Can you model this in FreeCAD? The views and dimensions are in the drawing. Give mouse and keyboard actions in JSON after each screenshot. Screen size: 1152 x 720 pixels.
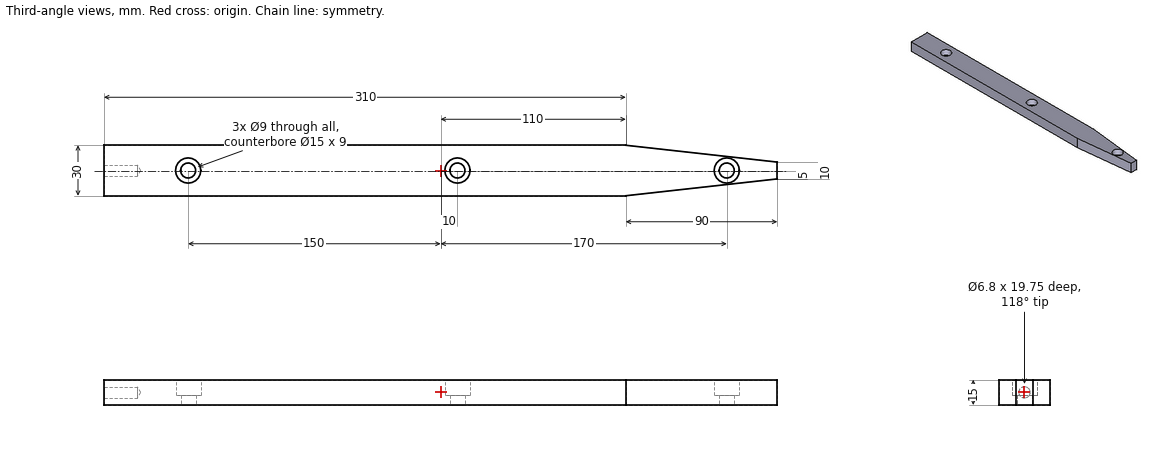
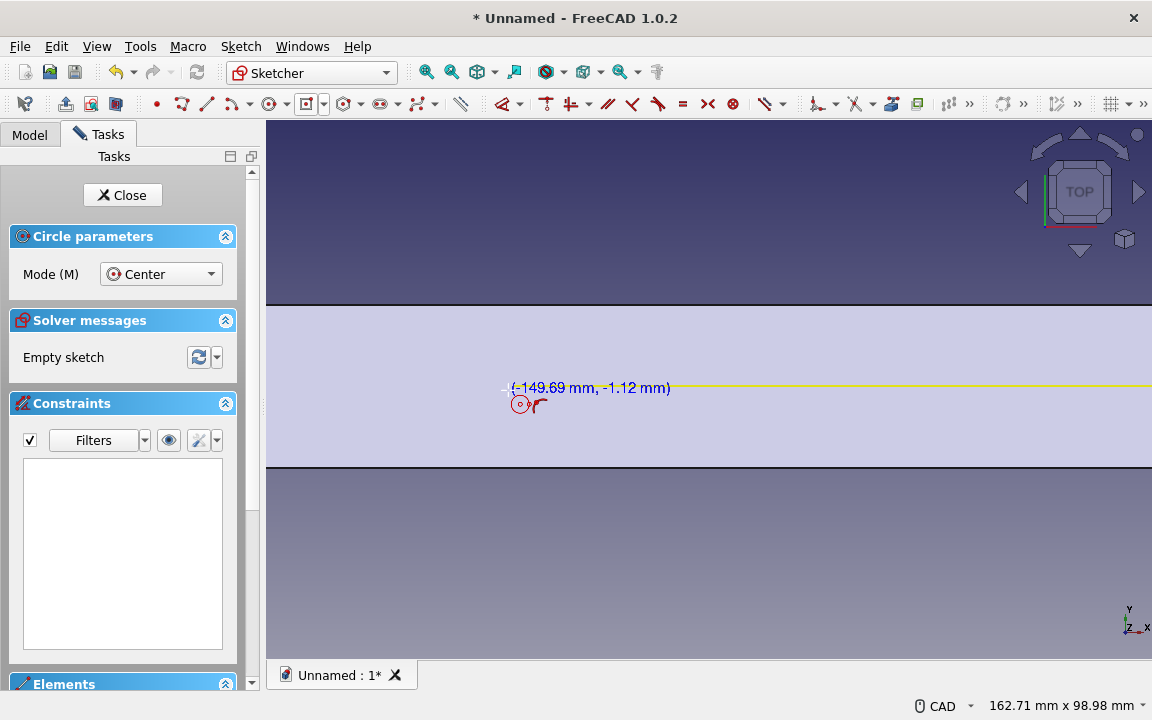
{"action": "scroll", "coordinate": [323, 391], "scroll_direction": "down", "scroll_amount": 6}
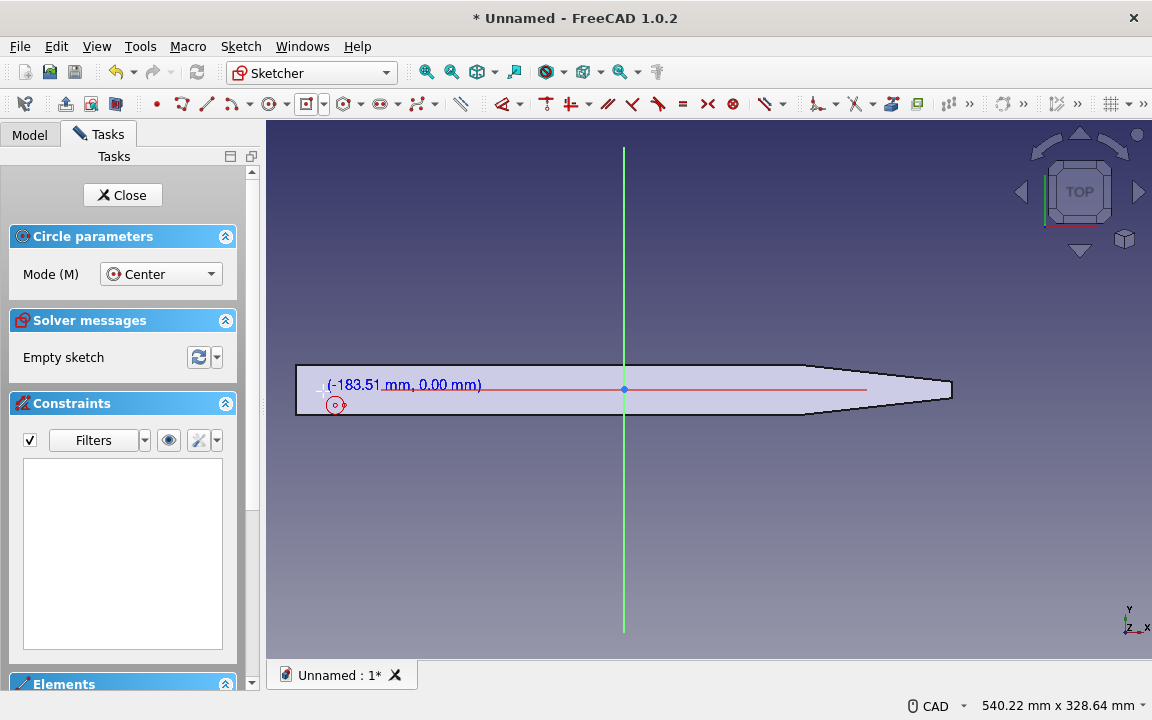
{"action": "left_click", "coordinate": [378, 390]}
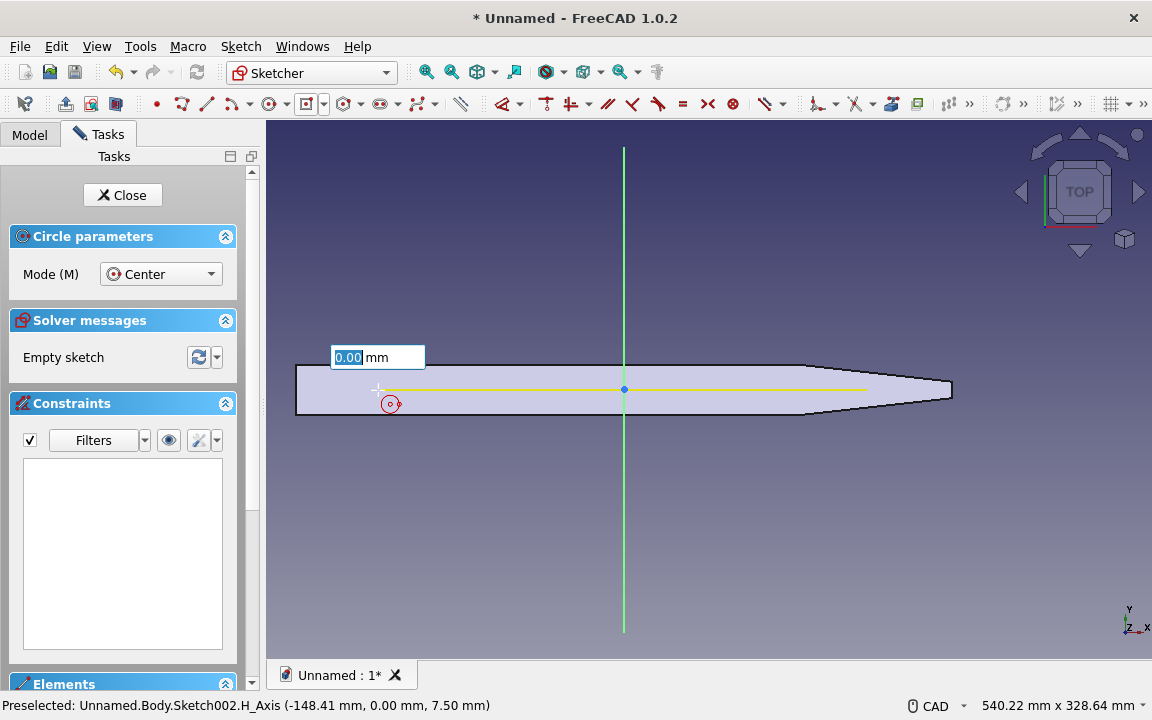
{"action": "scroll", "coordinate": [375, 397], "scroll_direction": "up", "scroll_amount": 5}
{"action": "mouse_move", "coordinate": [376, 396]}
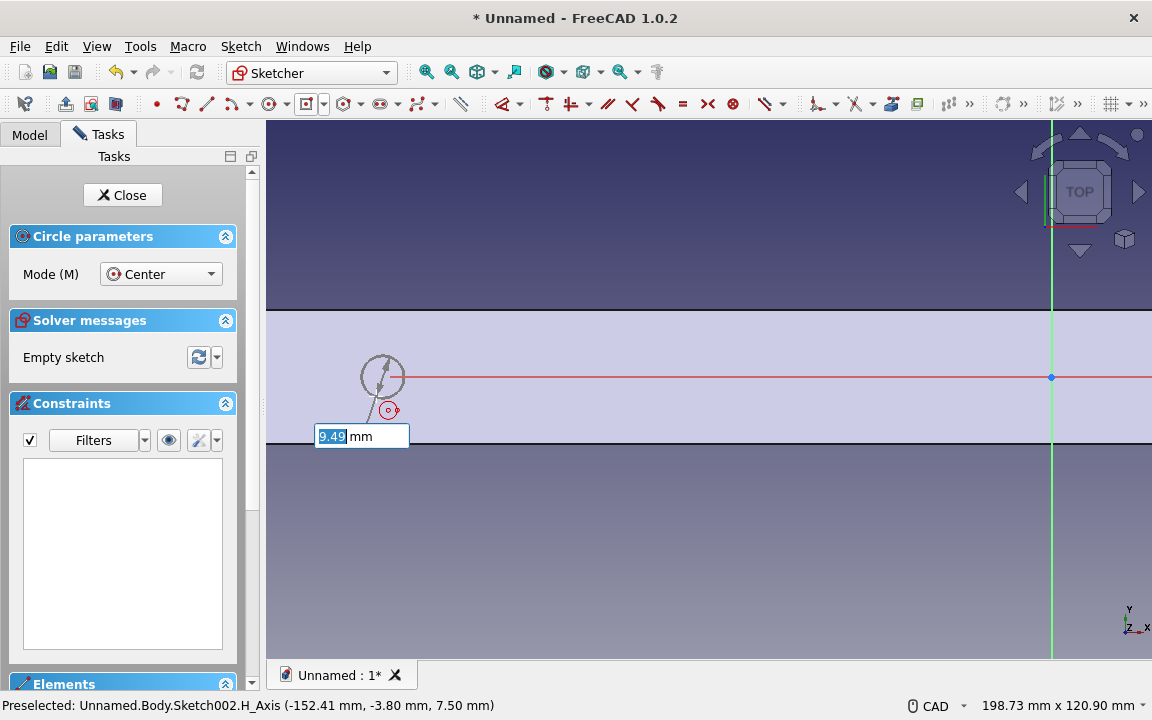
{"action": "type", "text": "9"}
{"action": "key", "text": "Return"}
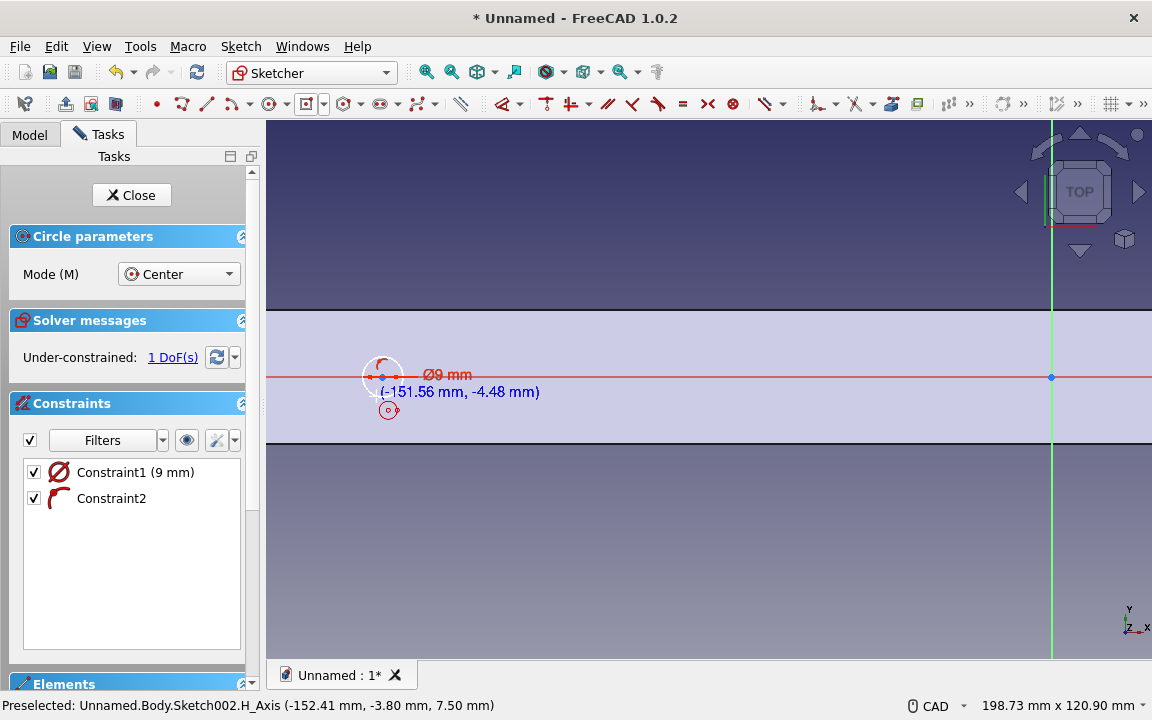
{"action": "scroll", "coordinate": [375, 397], "scroll_direction": "down", "scroll_amount": 5}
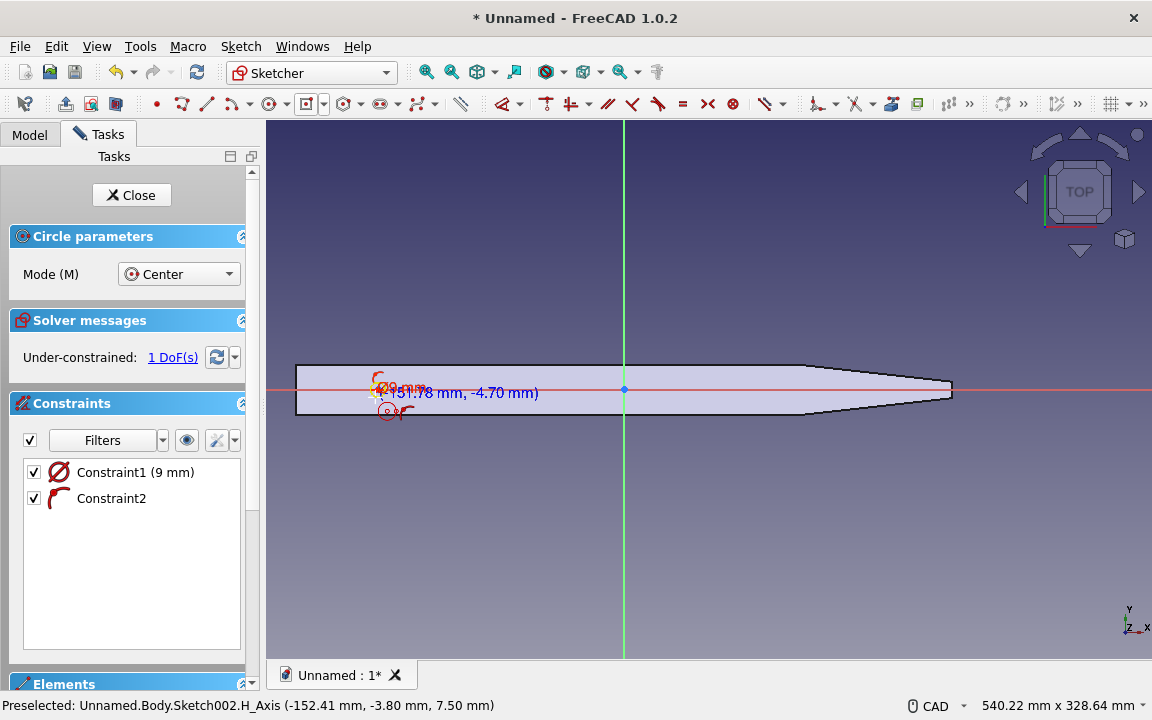
{"action": "scroll", "coordinate": [903, 390], "scroll_direction": "up", "scroll_amount": 6}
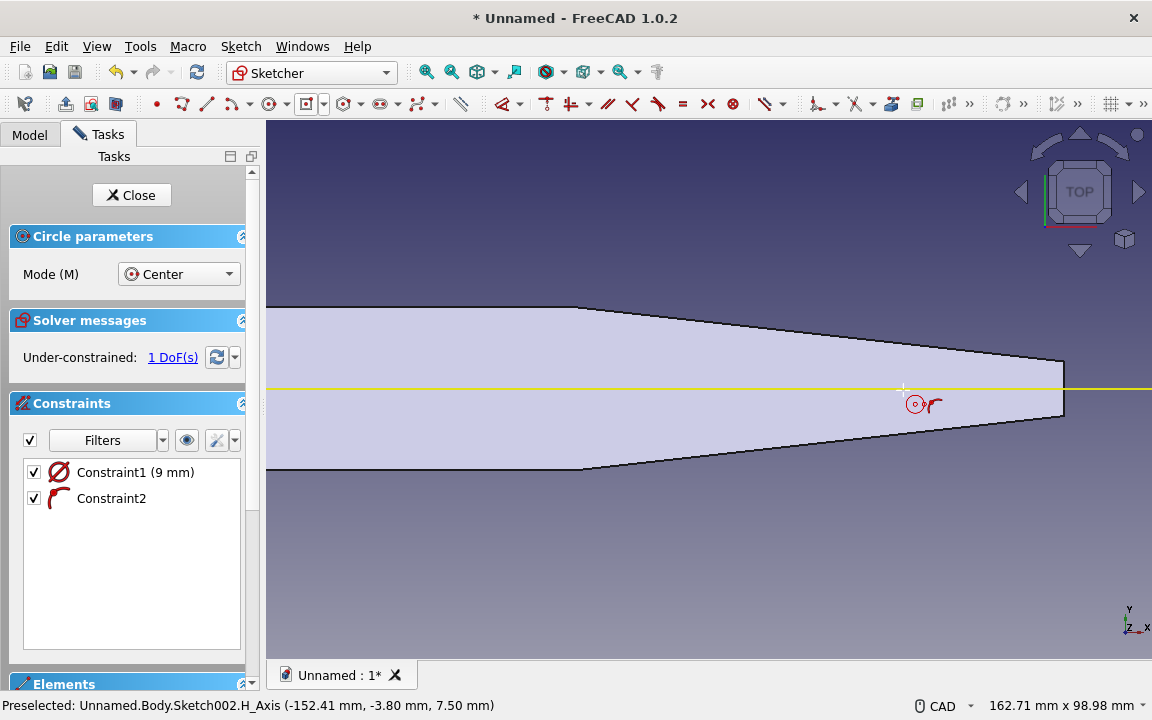
{"action": "scroll", "coordinate": [904, 390], "scroll_direction": "down", "scroll_amount": 6}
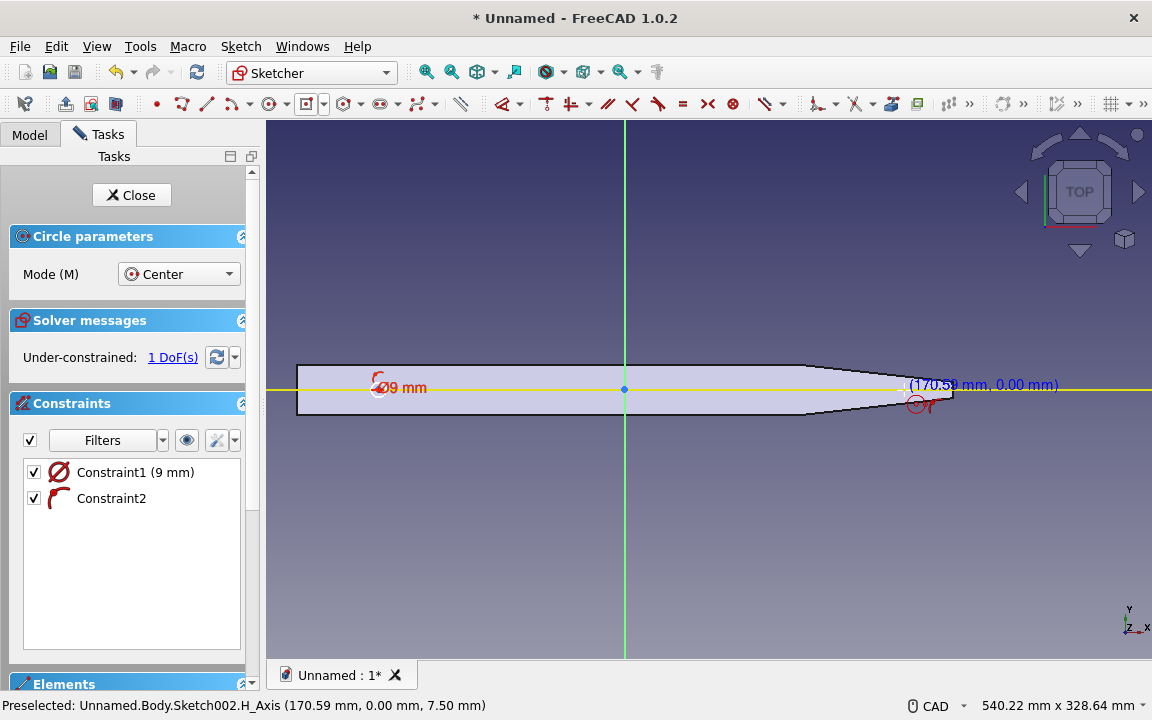
{"action": "left_click", "coordinate": [904, 390]}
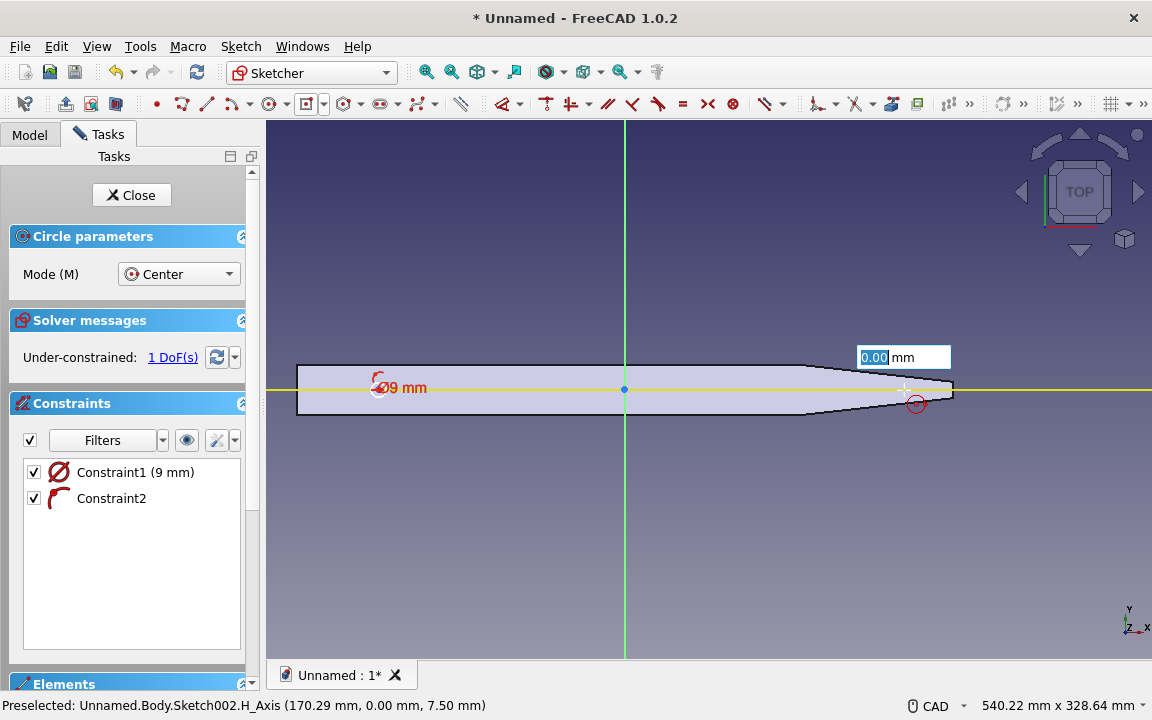
{"action": "scroll", "coordinate": [901, 397], "scroll_direction": "up", "scroll_amount": 5}
{"action": "mouse_move", "coordinate": [900, 396]}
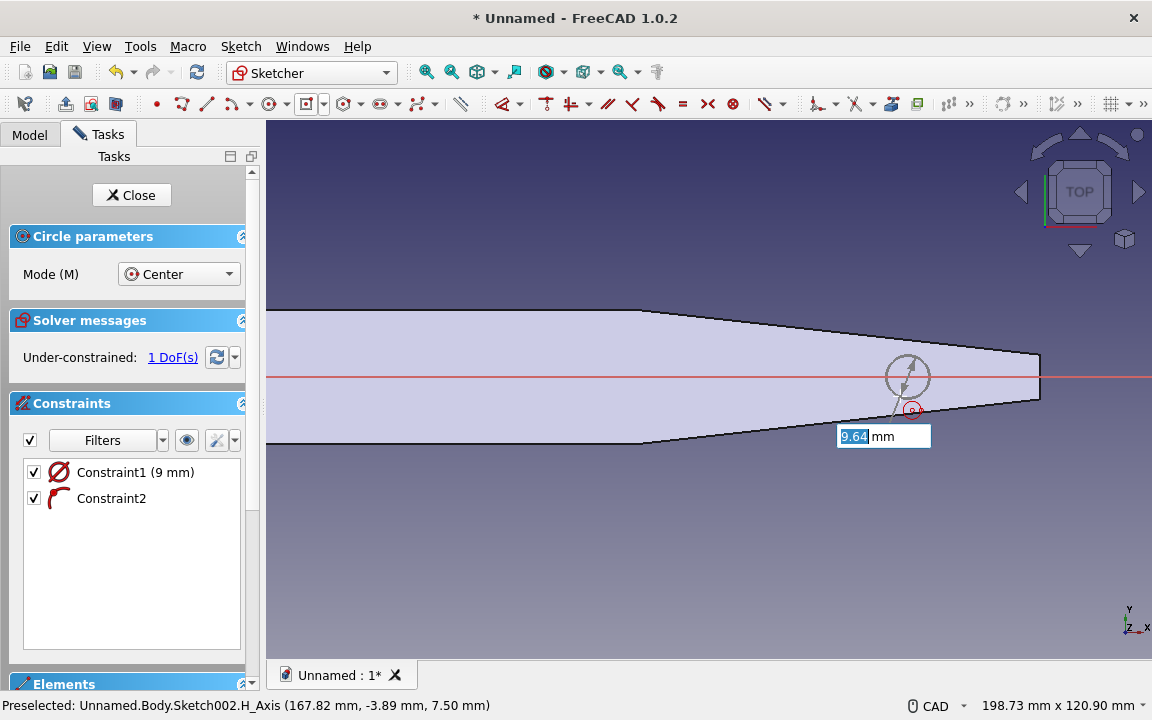
{"action": "type", "text": "9"}
{"action": "key", "text": "Return"}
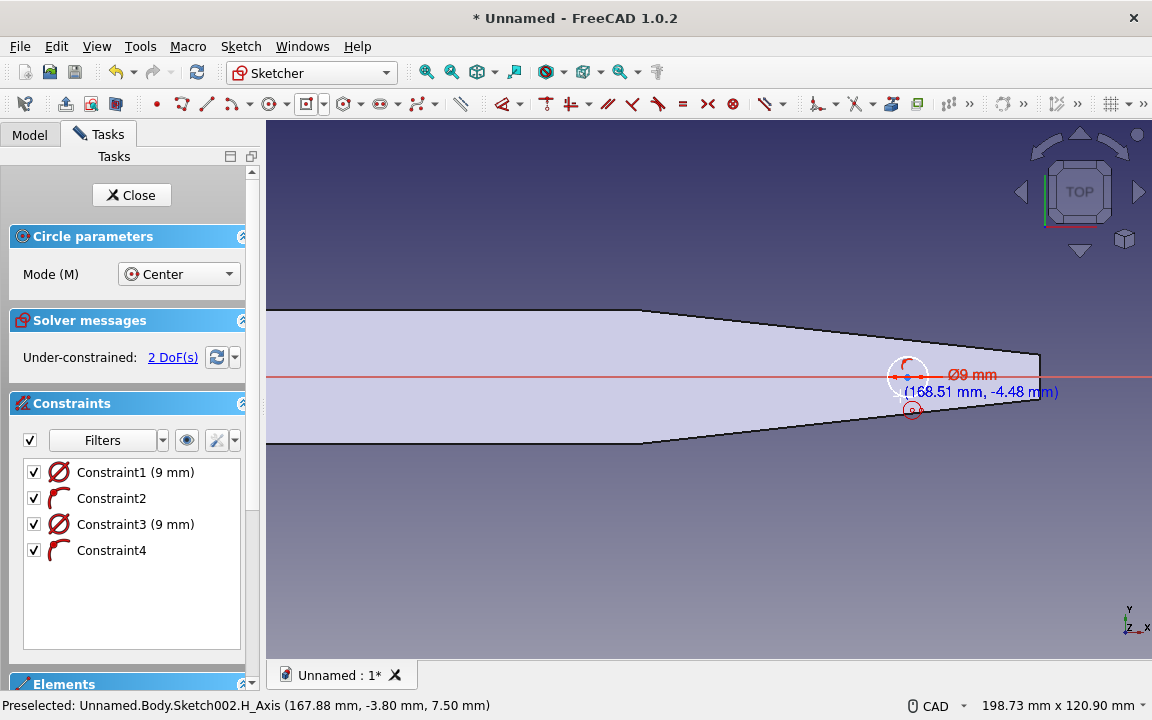
{"action": "scroll", "coordinate": [901, 397], "scroll_direction": "down", "scroll_amount": 5}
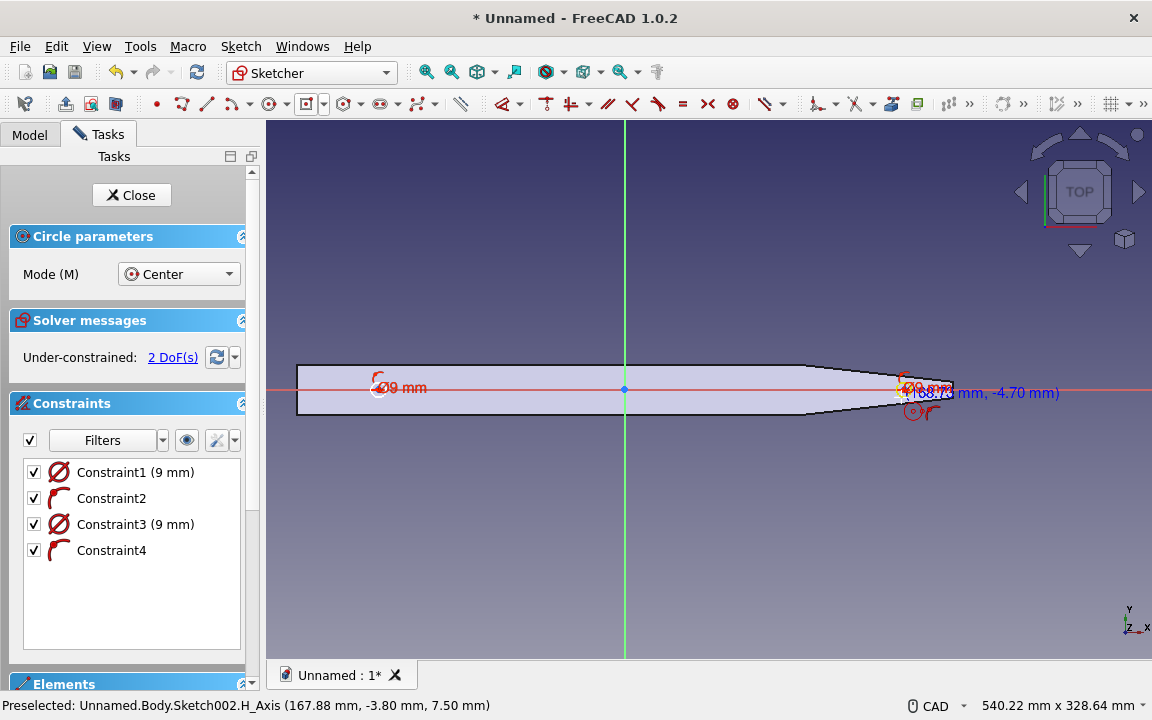
{"action": "scroll", "coordinate": [641, 390], "scroll_direction": "up", "scroll_amount": 6}